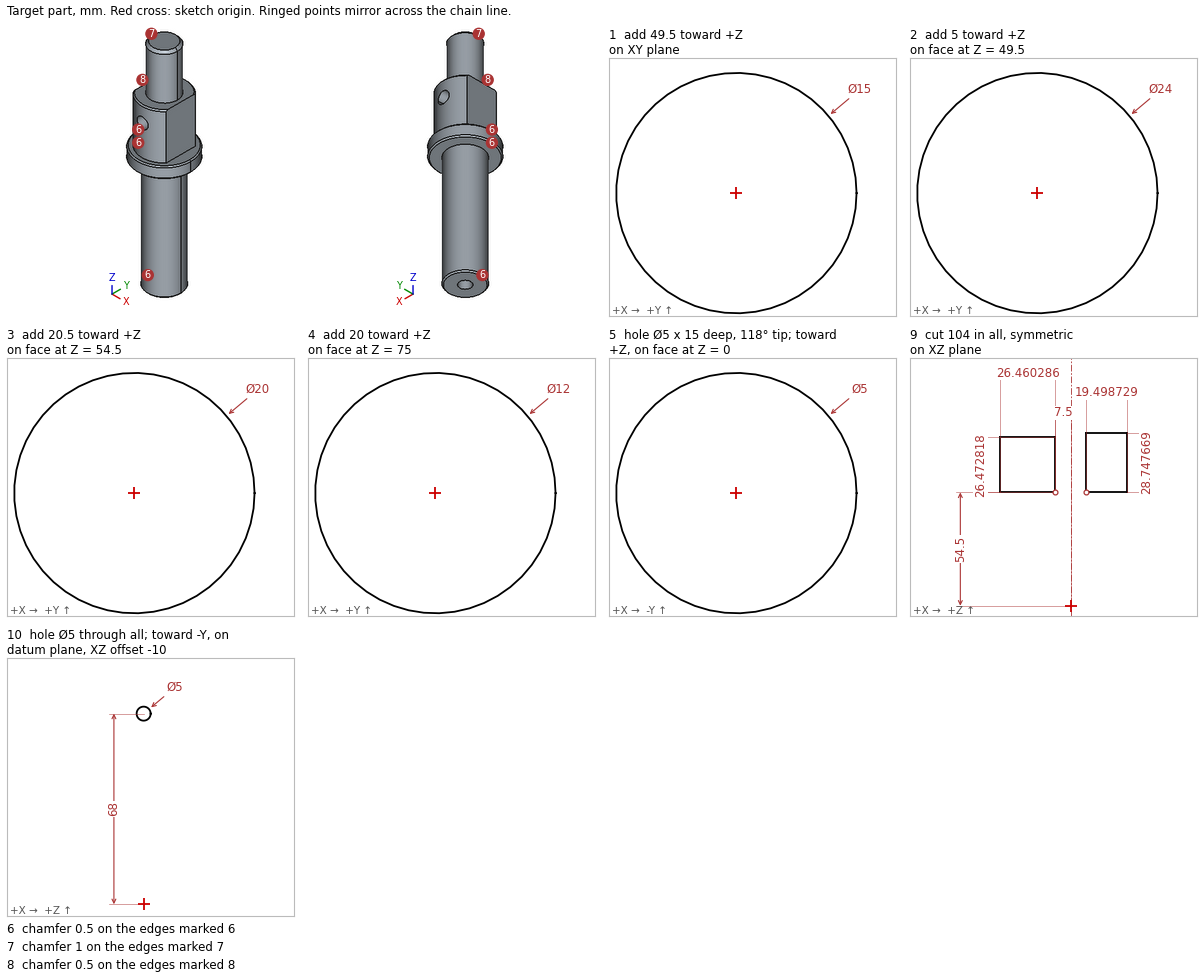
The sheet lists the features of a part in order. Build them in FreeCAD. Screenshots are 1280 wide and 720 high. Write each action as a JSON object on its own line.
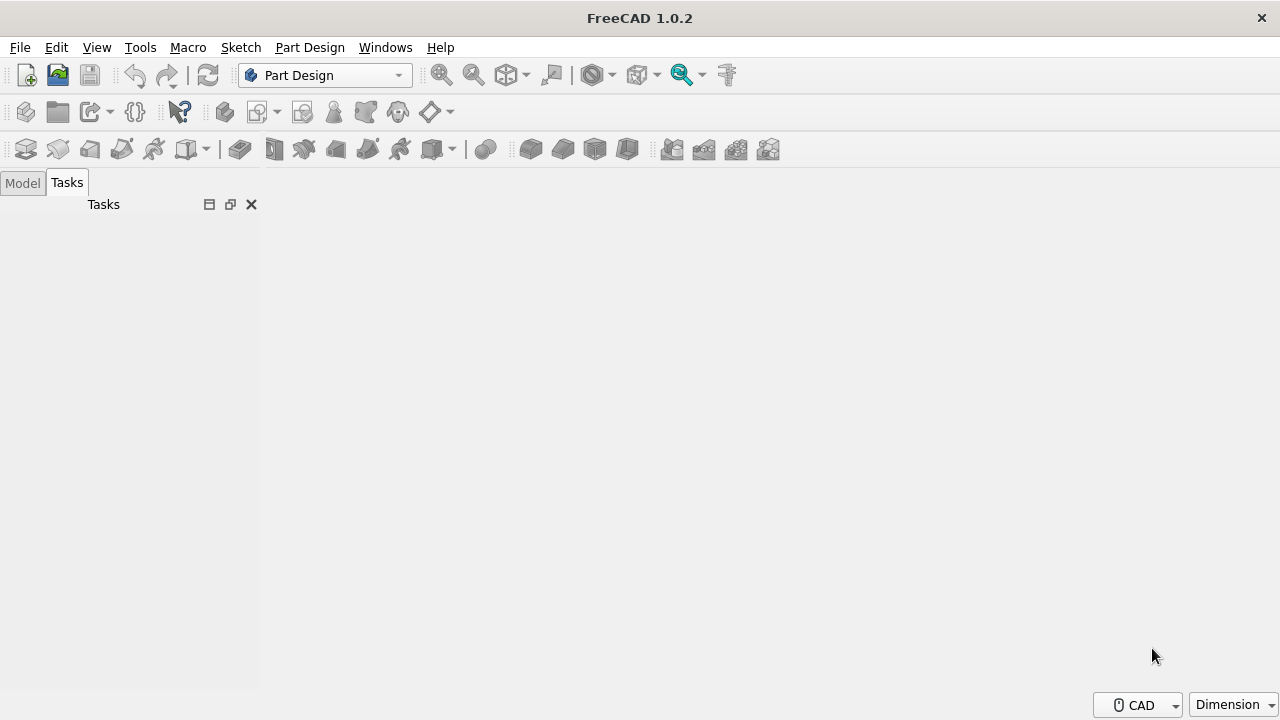
{"action": "key", "text": "ctrl+n"}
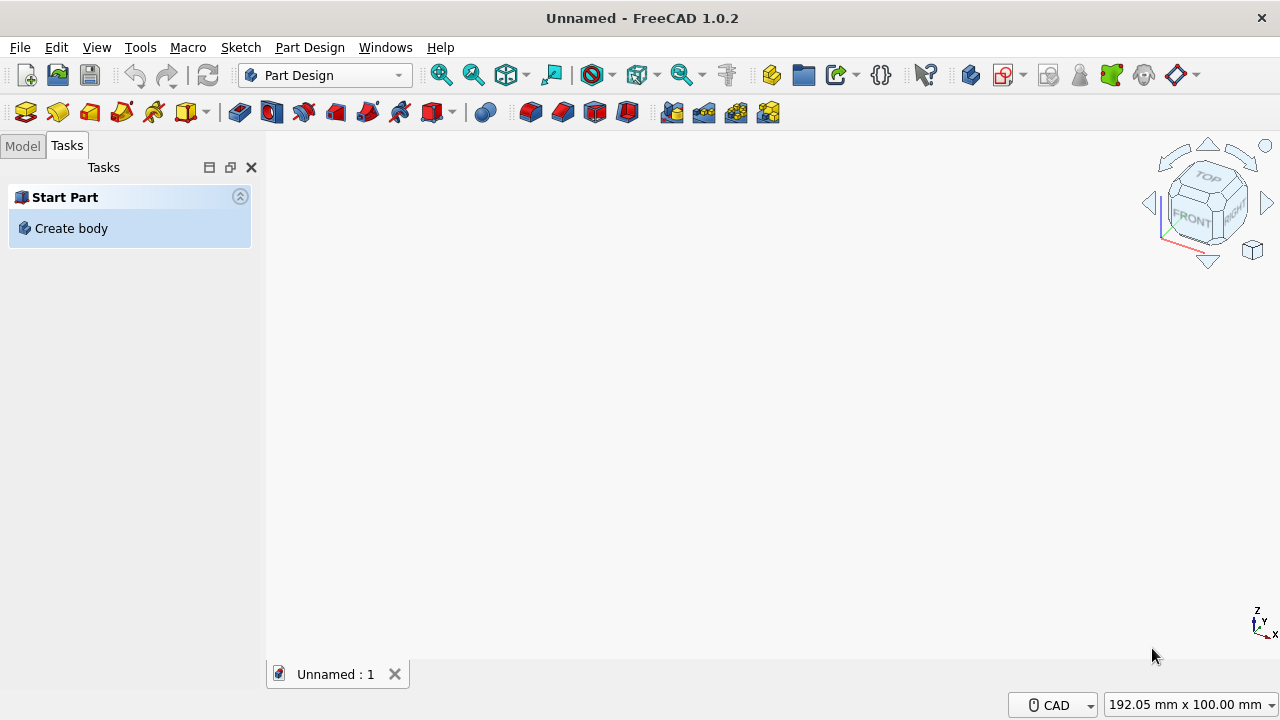
{"action": "left_click", "coordinate": [1004, 76]}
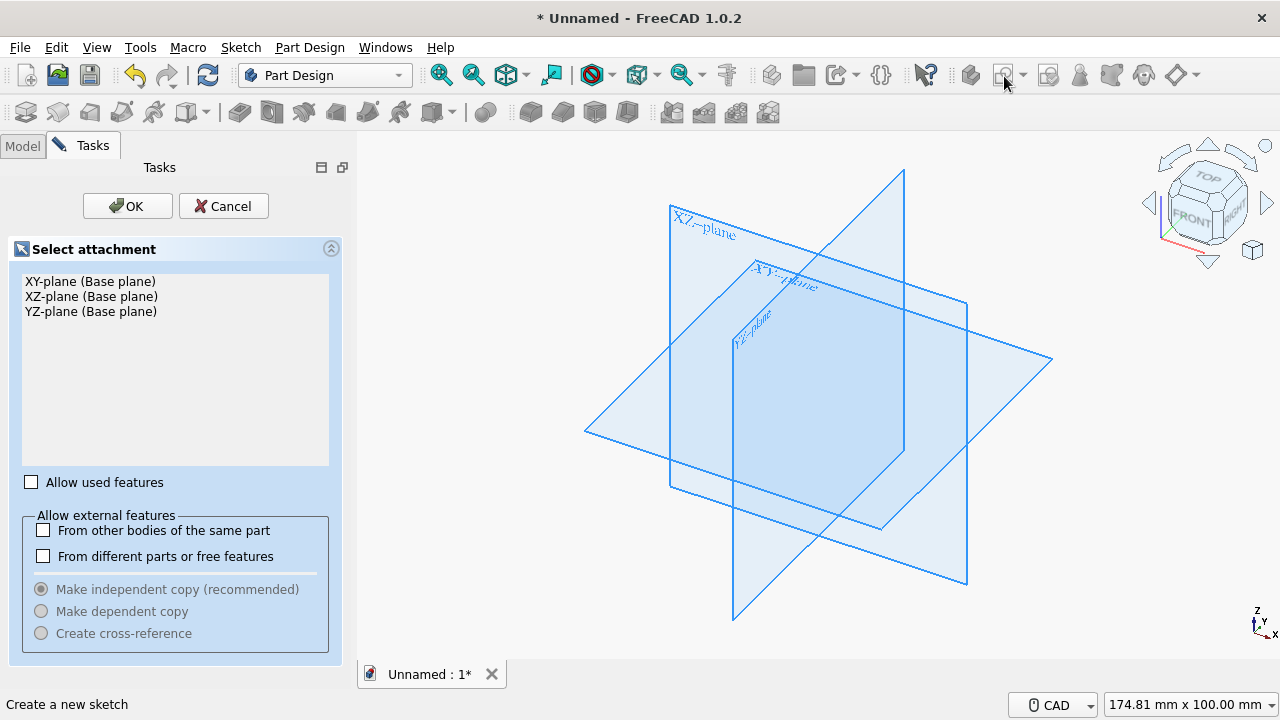
{"action": "left_click", "coordinate": [82, 282]}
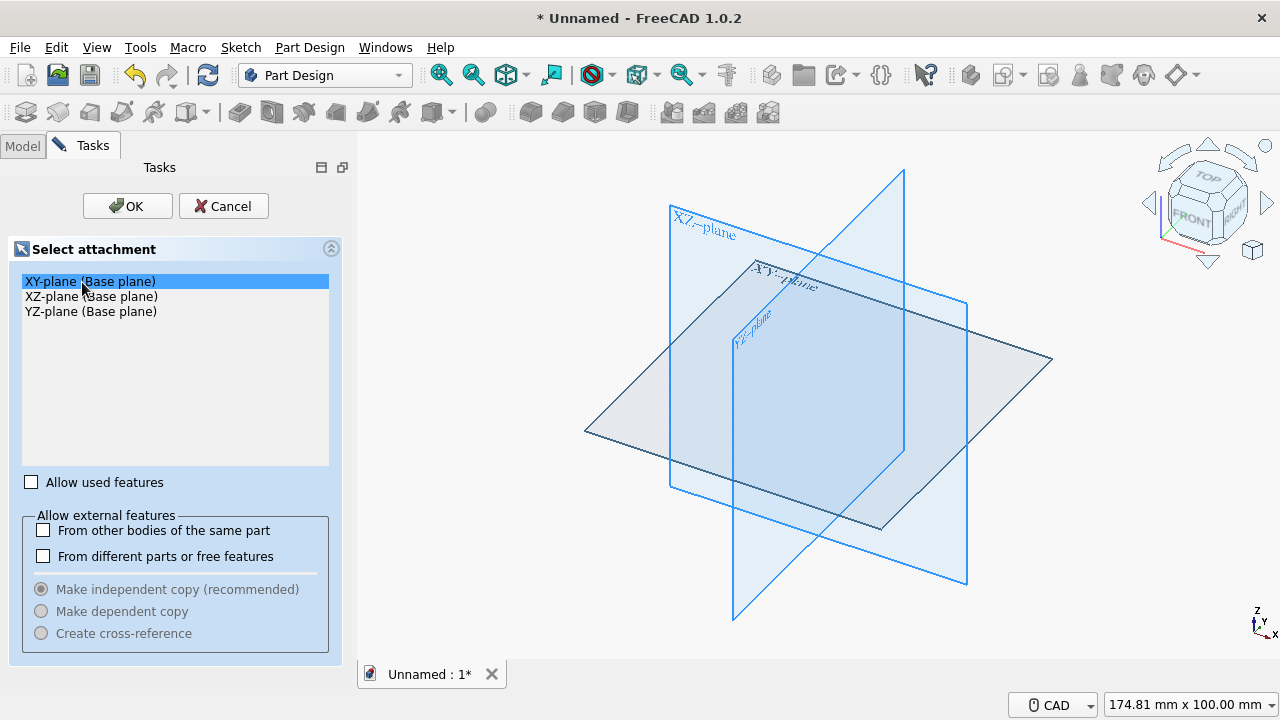
{"action": "left_click", "coordinate": [128, 206]}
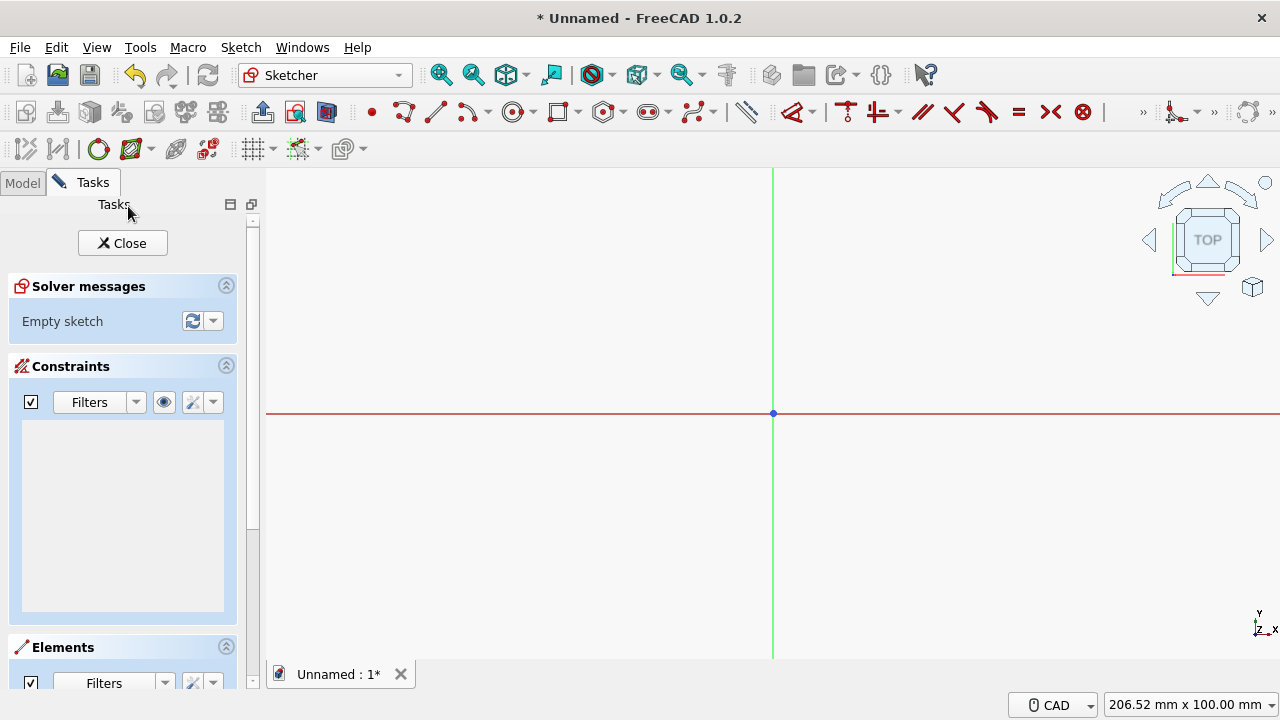
{"action": "scroll", "coordinate": [795, 414], "scroll_direction": "up", "scroll_amount": 7}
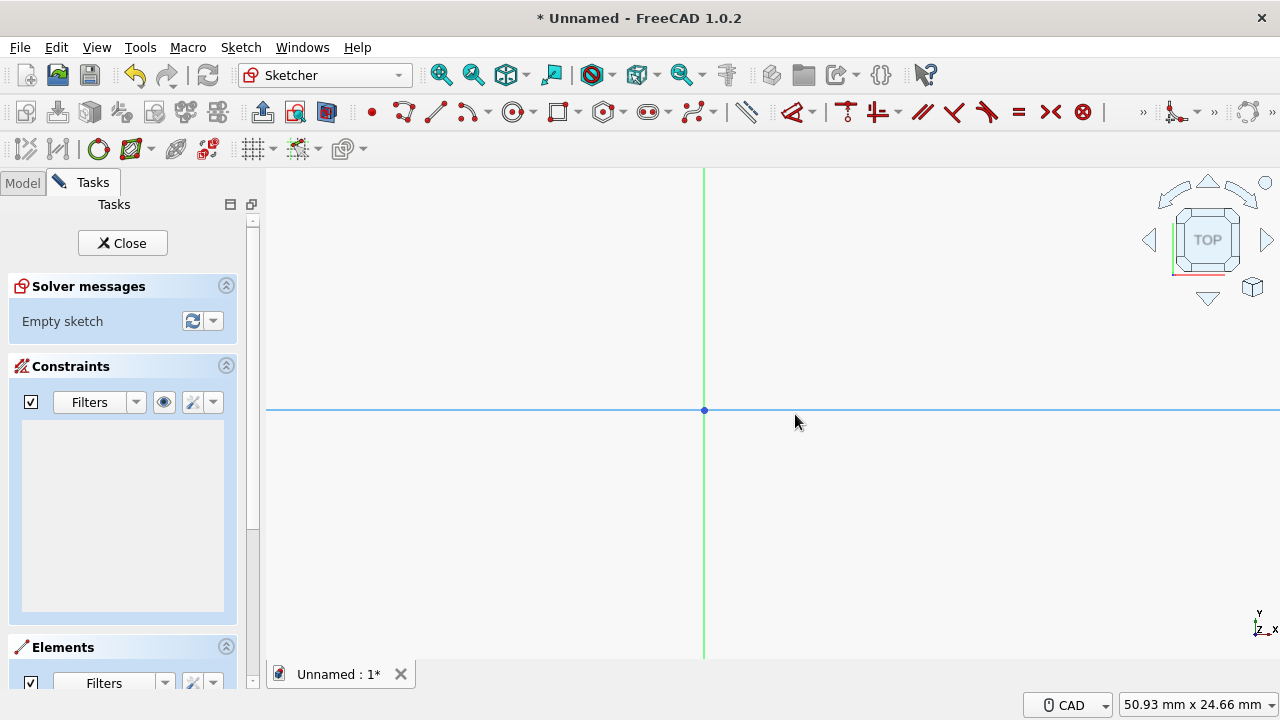
{"action": "key", "text": "g c"}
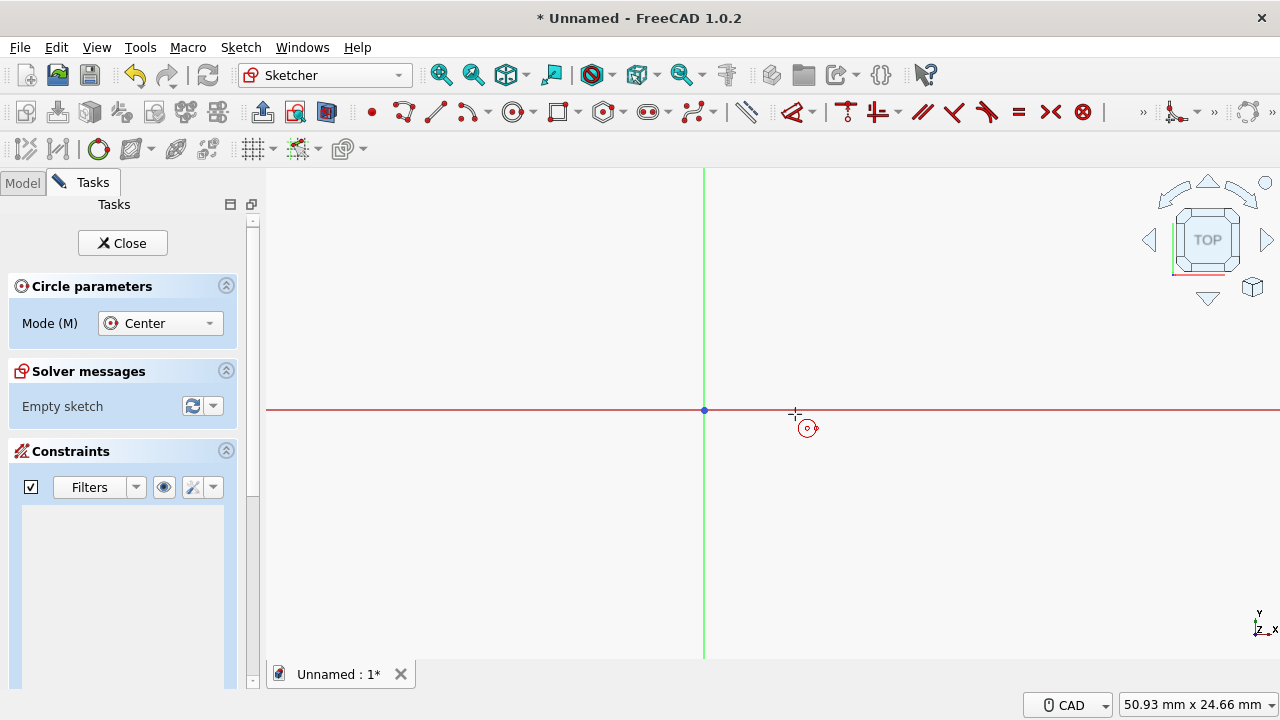
{"action": "left_click", "coordinate": [704, 410]}
{"action": "mouse_move", "coordinate": [810, 305]}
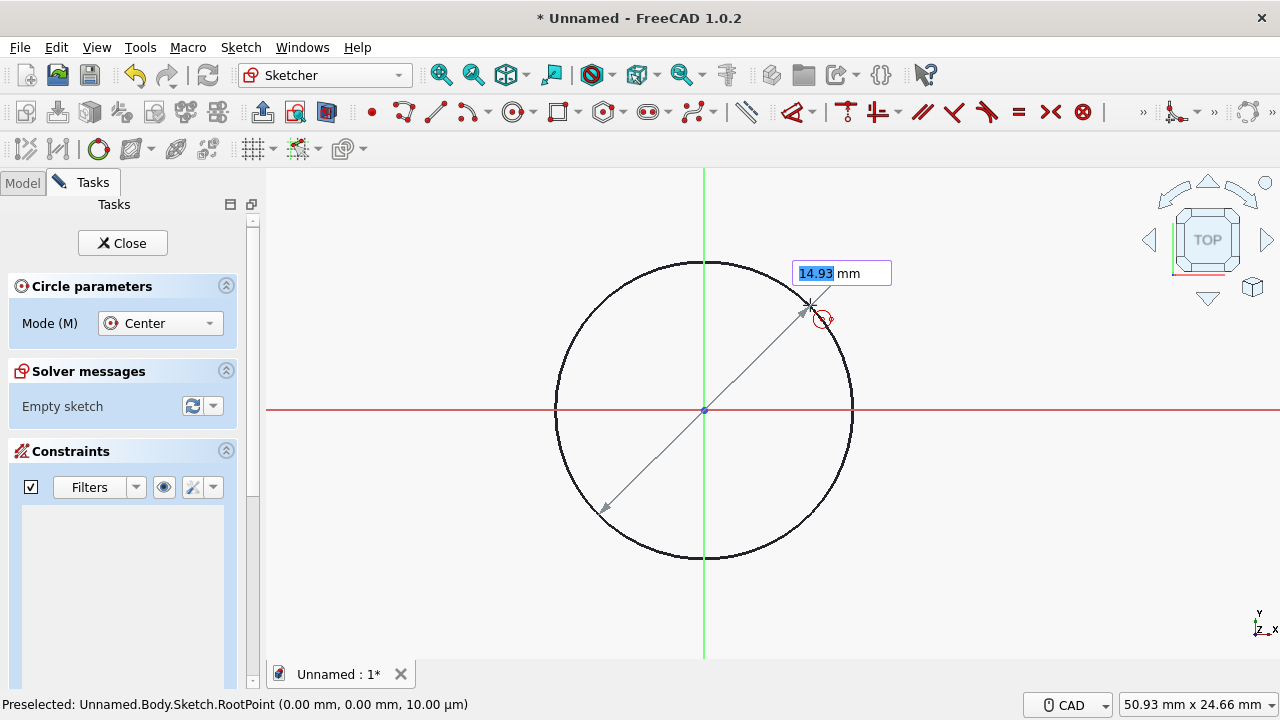
{"action": "type", "text": "15"}
{"action": "key", "text": "Return"}
{"action": "key", "text": "Escape"}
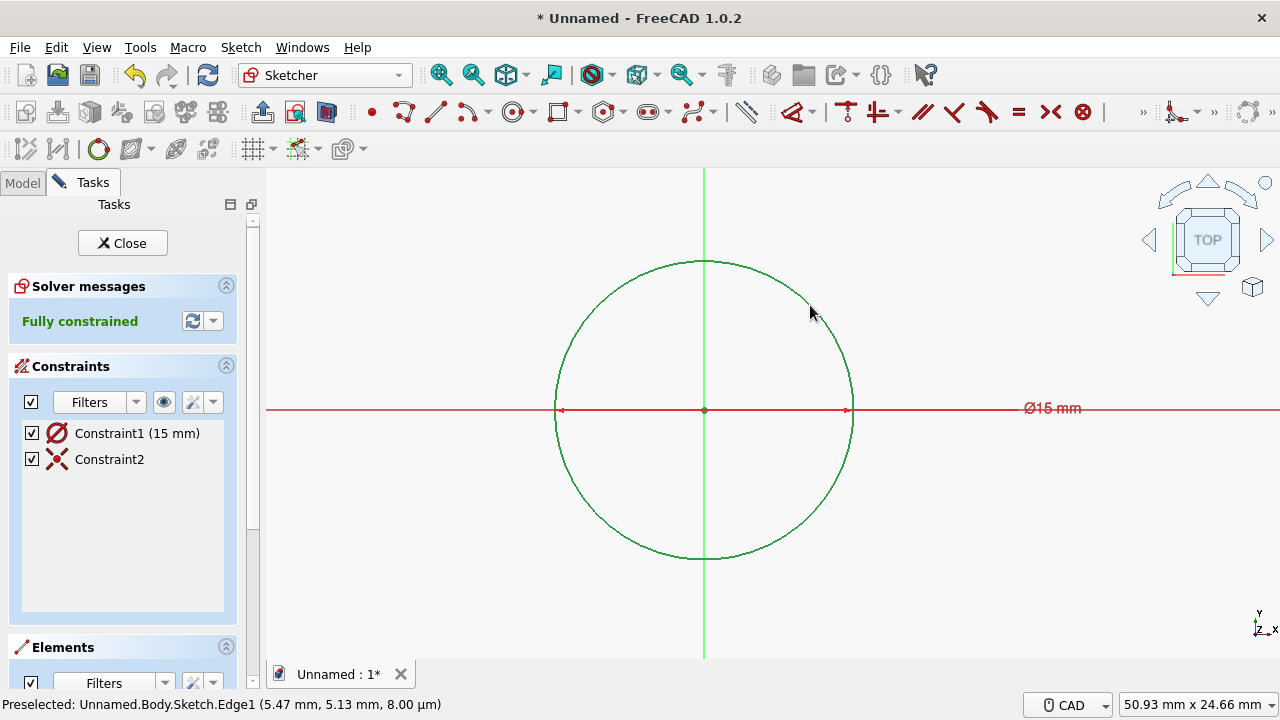
{"action": "left_click", "coordinate": [123, 243]}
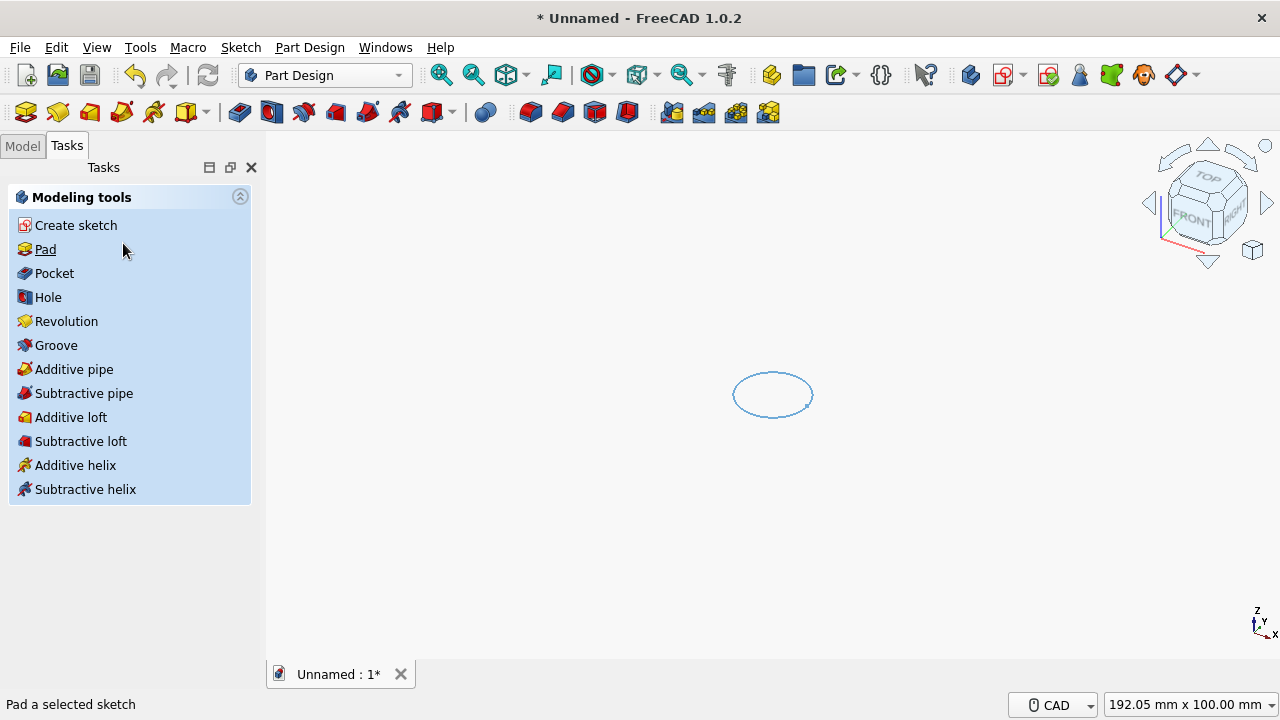
{"action": "left_click", "coordinate": [26, 112]}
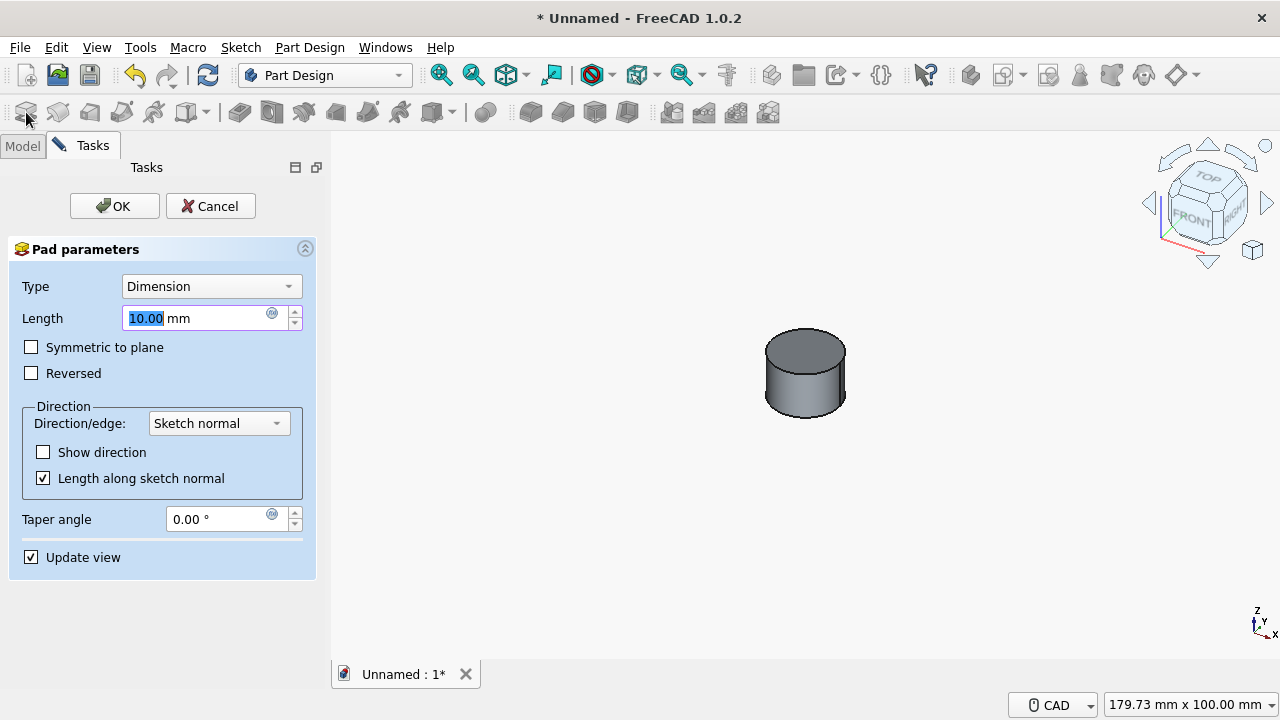
{"action": "type", "text": "49.5"}
{"action": "key", "text": "Tab"}